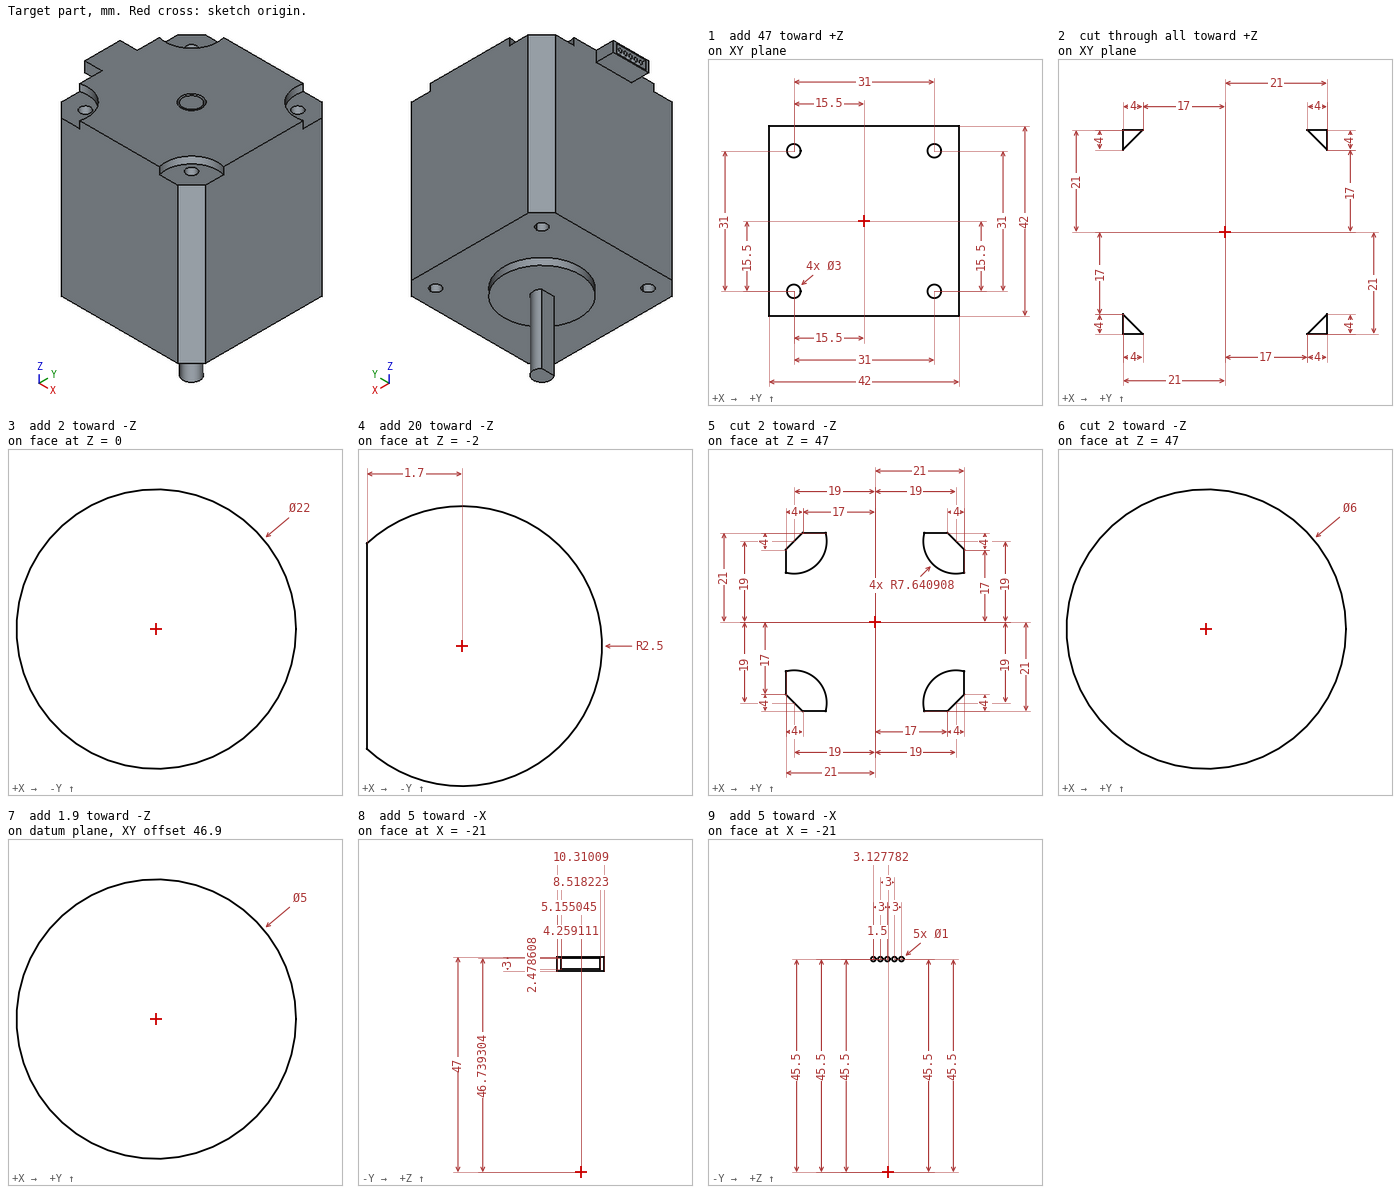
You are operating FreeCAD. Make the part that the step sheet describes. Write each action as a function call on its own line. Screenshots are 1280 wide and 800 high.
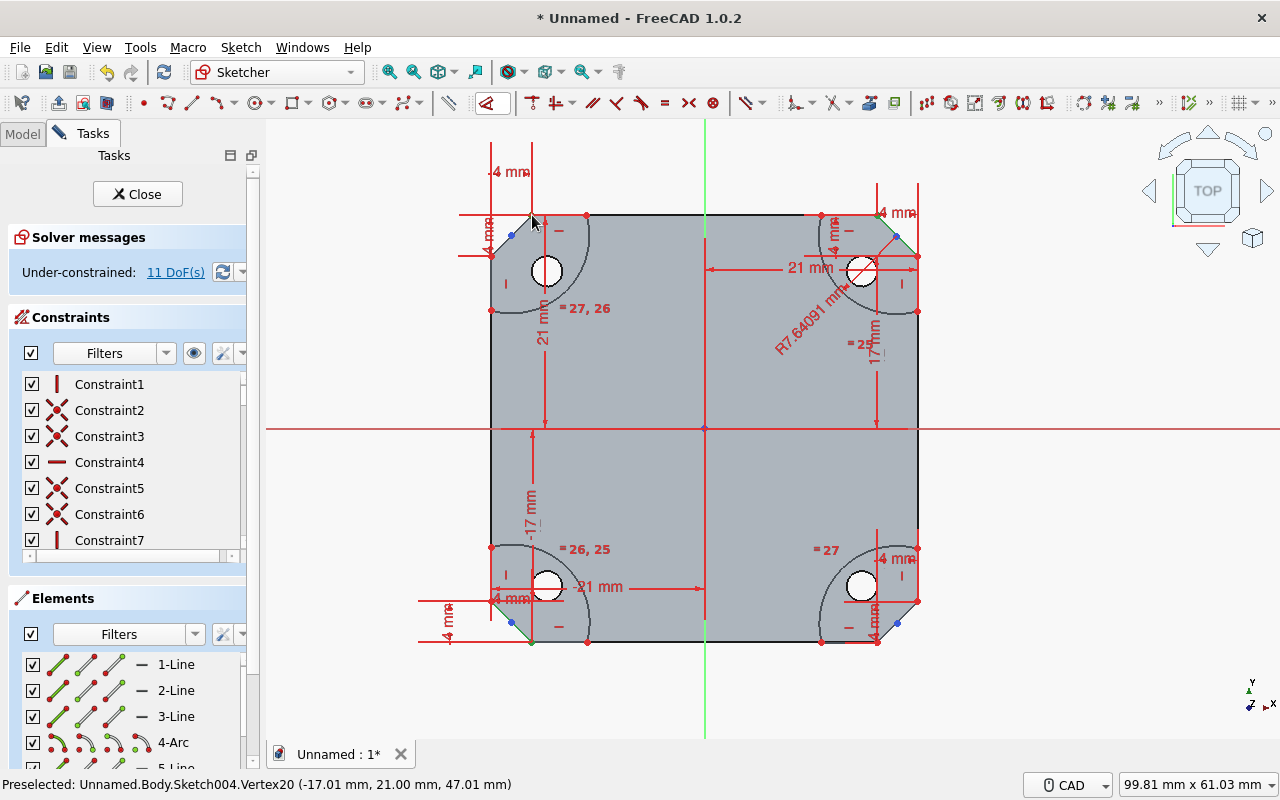
key(l)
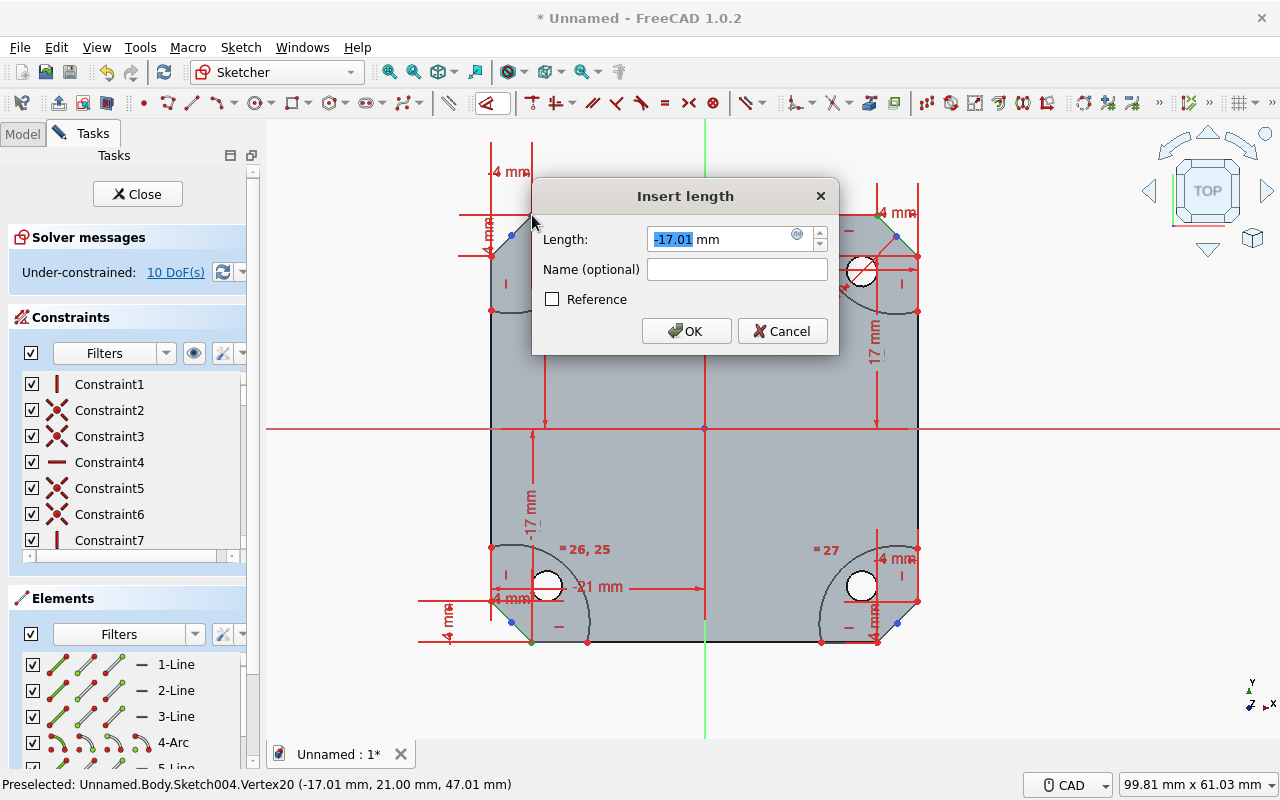
text(-17)
key(Return)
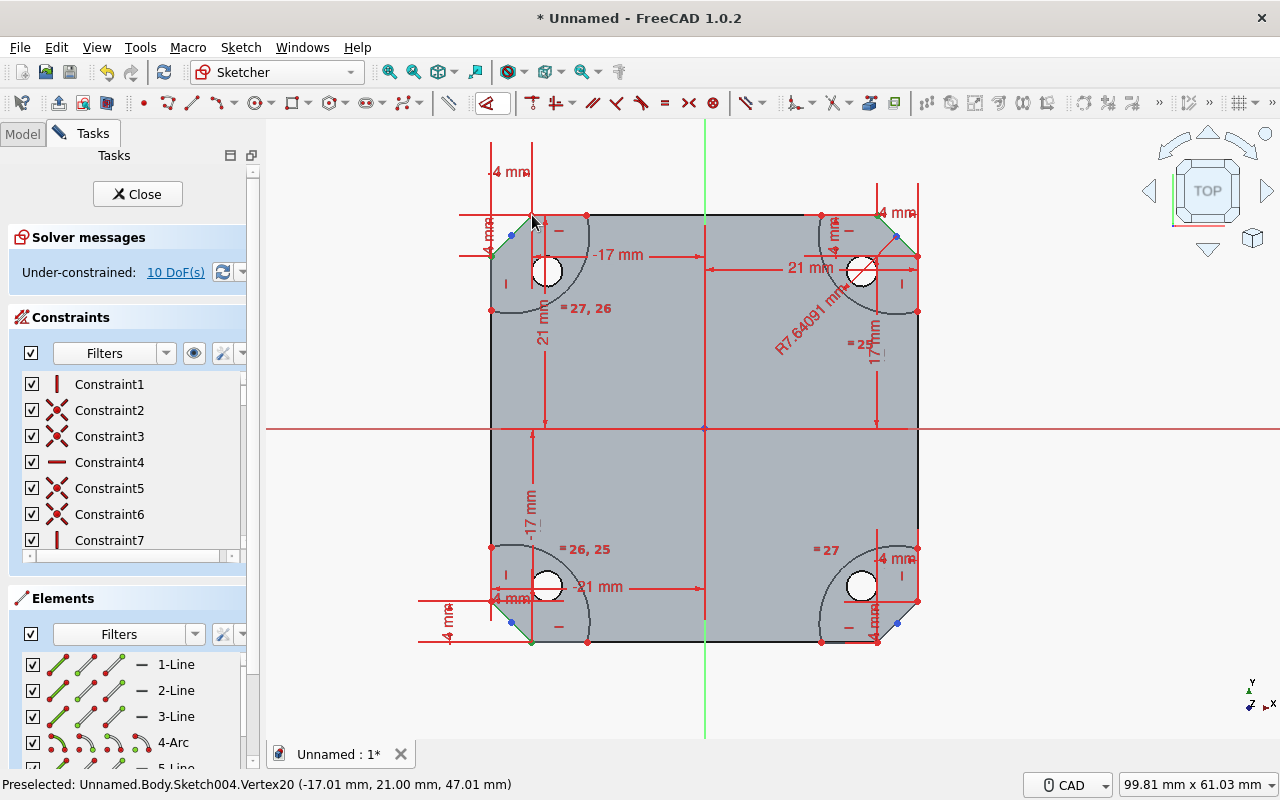
click(822, 643)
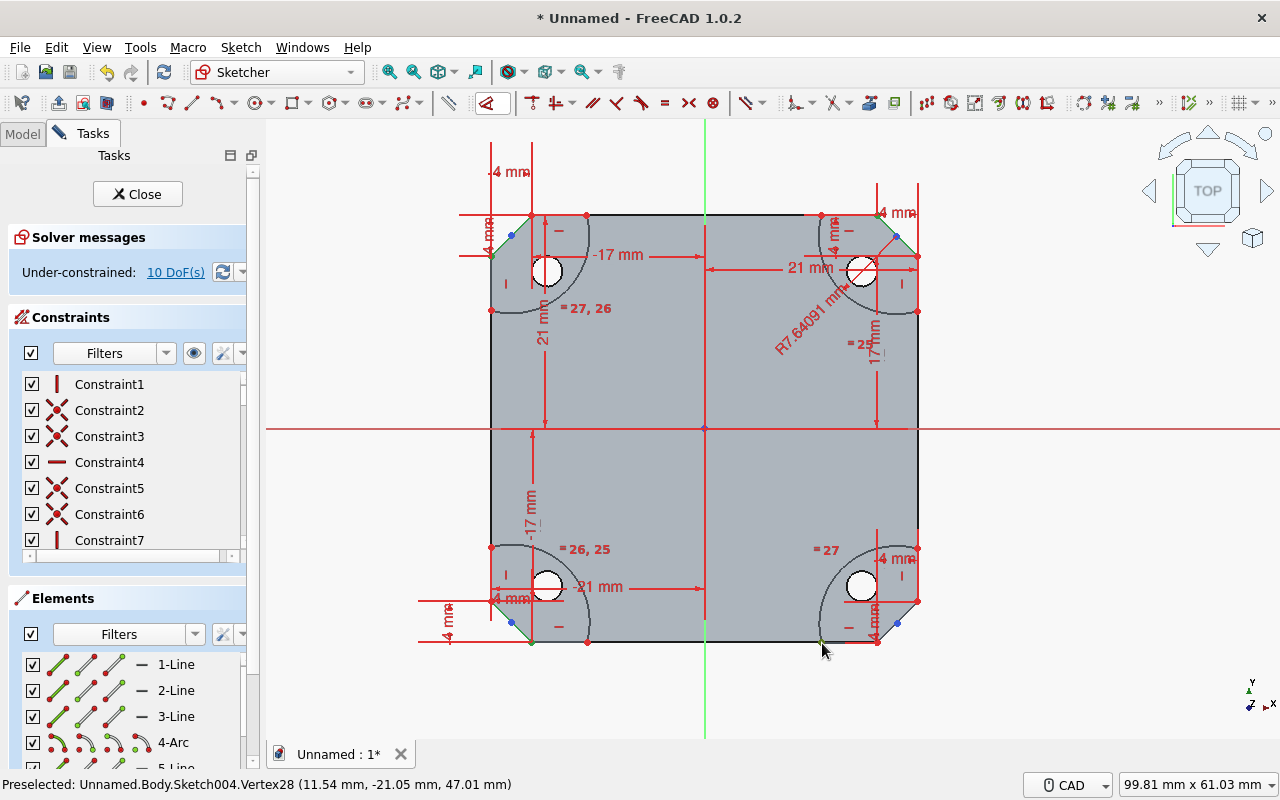
key(i)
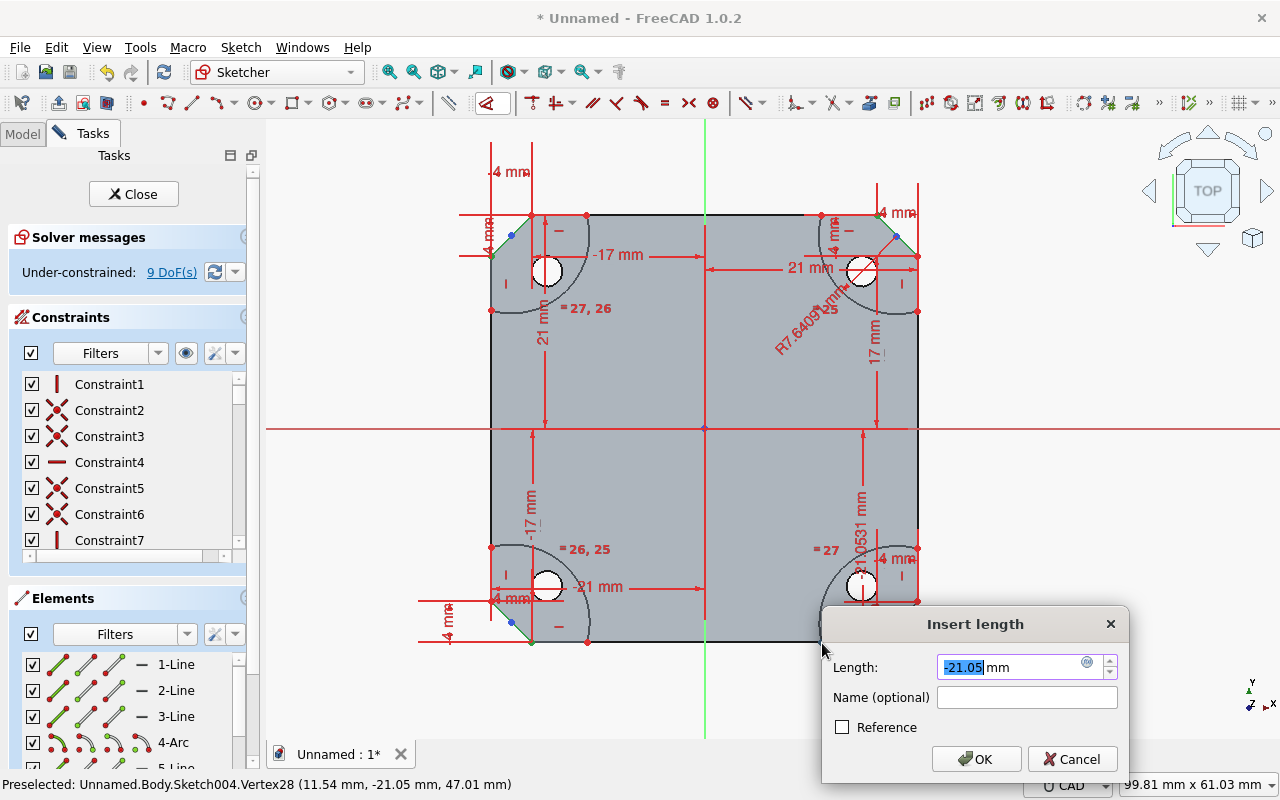
text(-21)
key(Return)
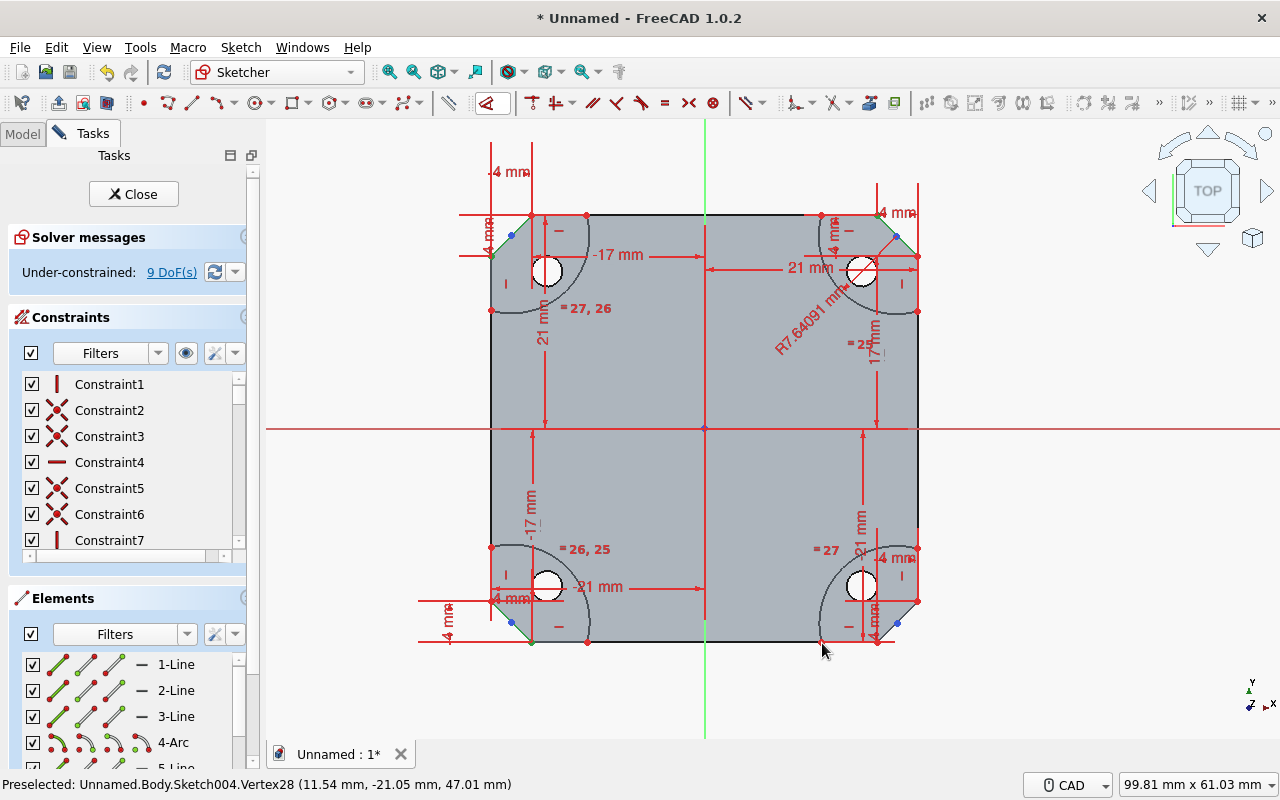
click(877, 642)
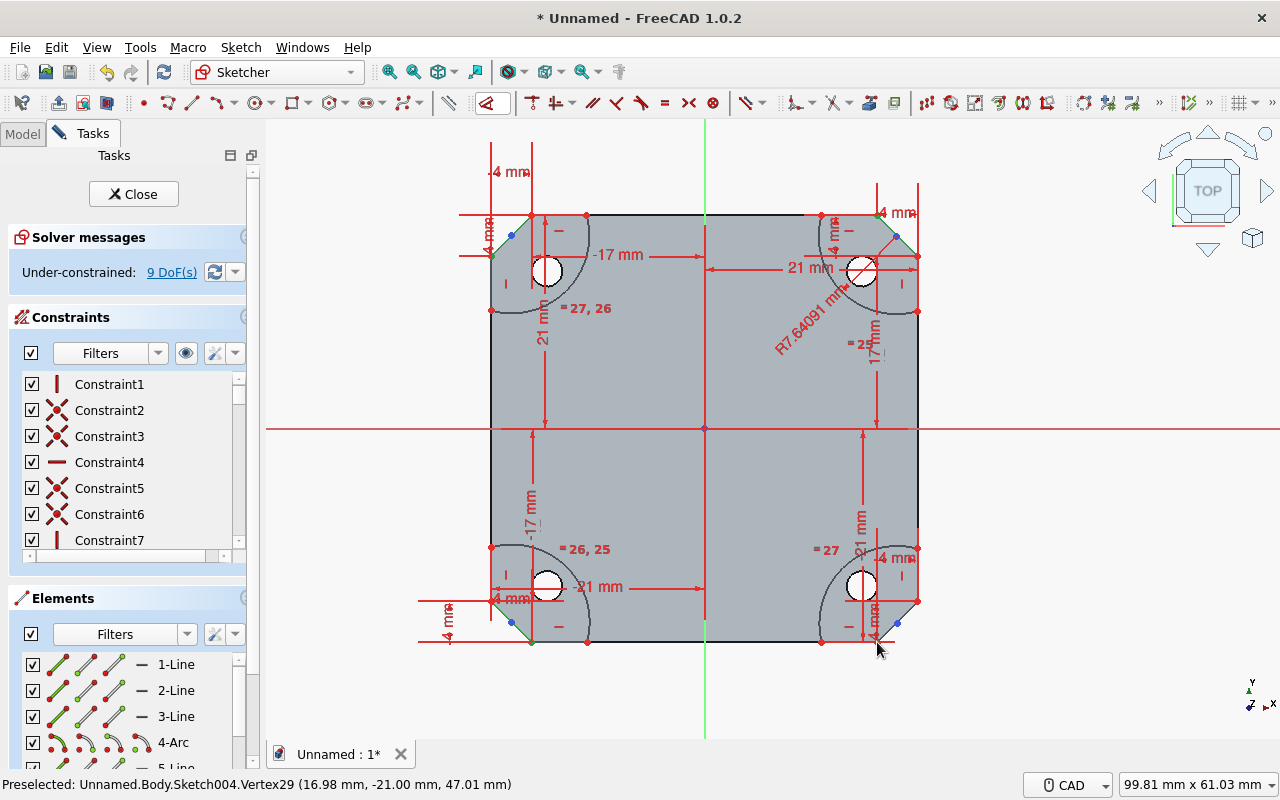
key(l)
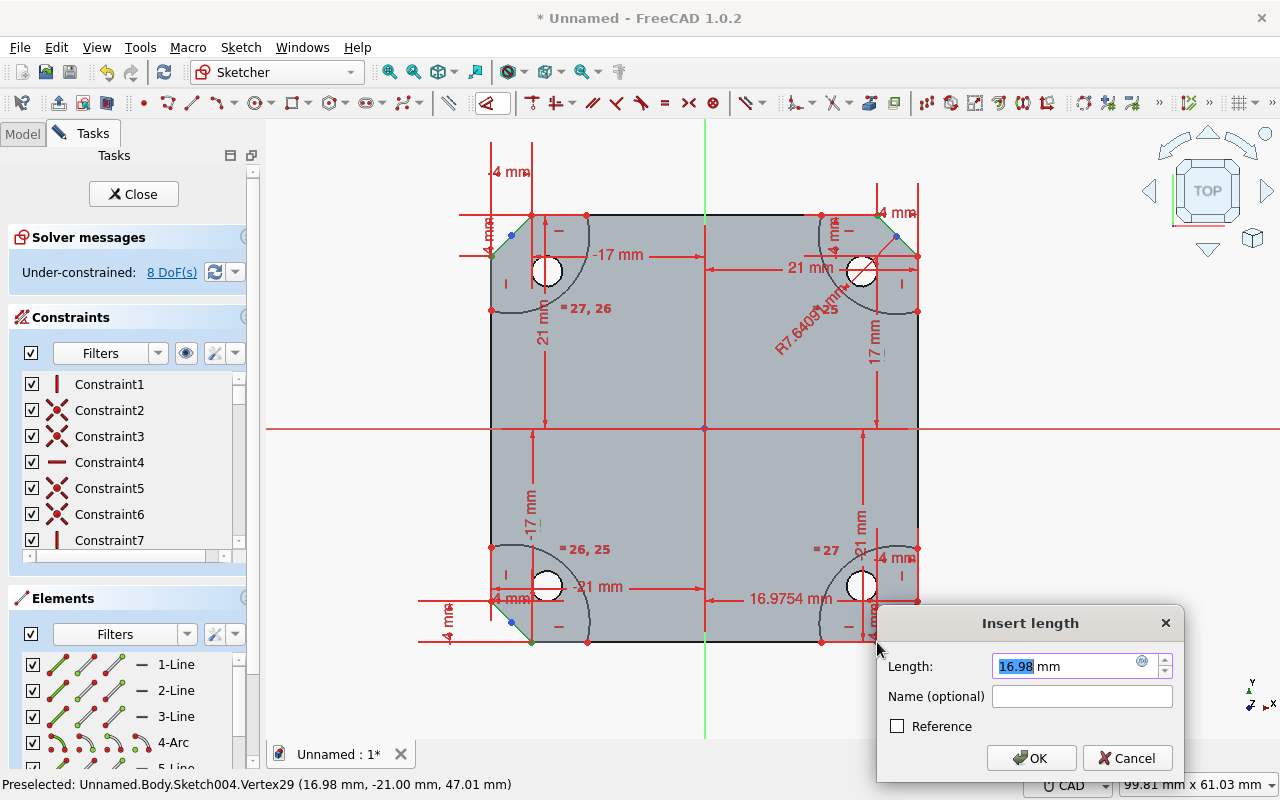
text(17)
key(Return)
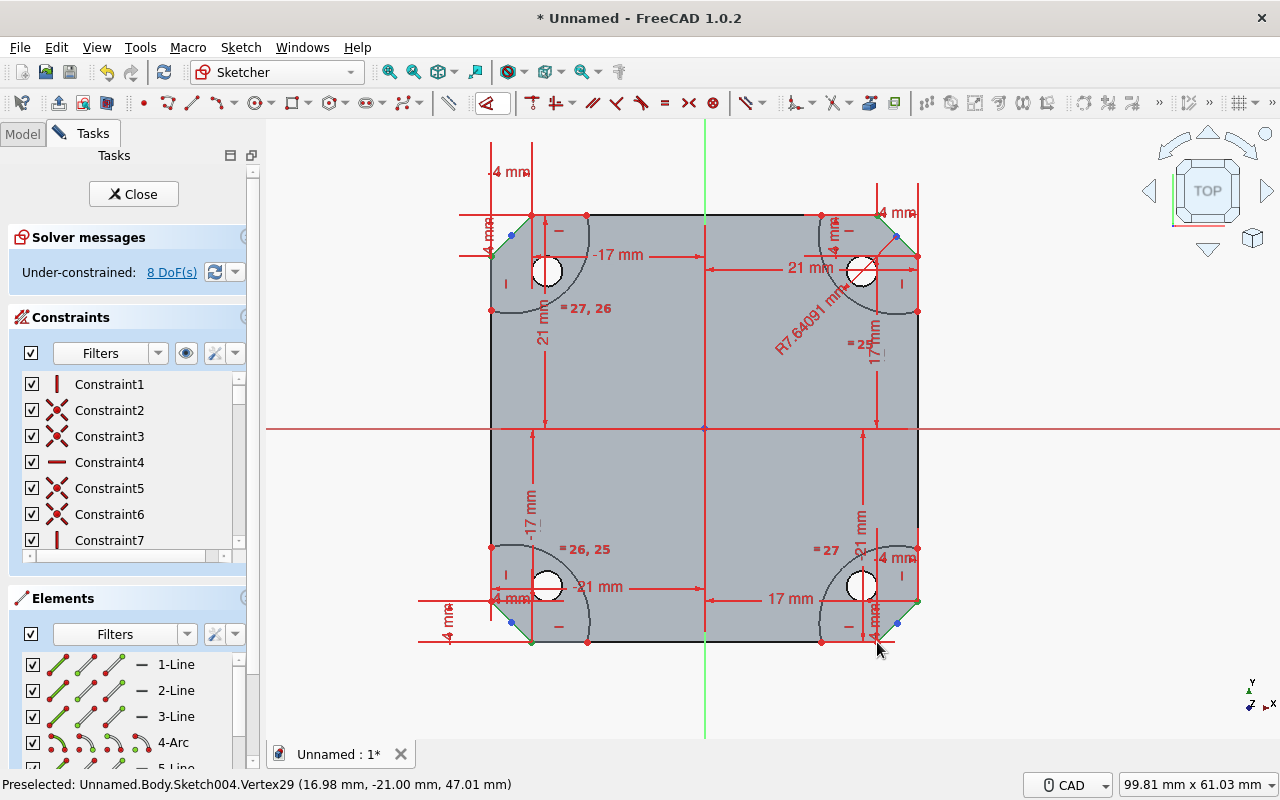
click(896, 236)